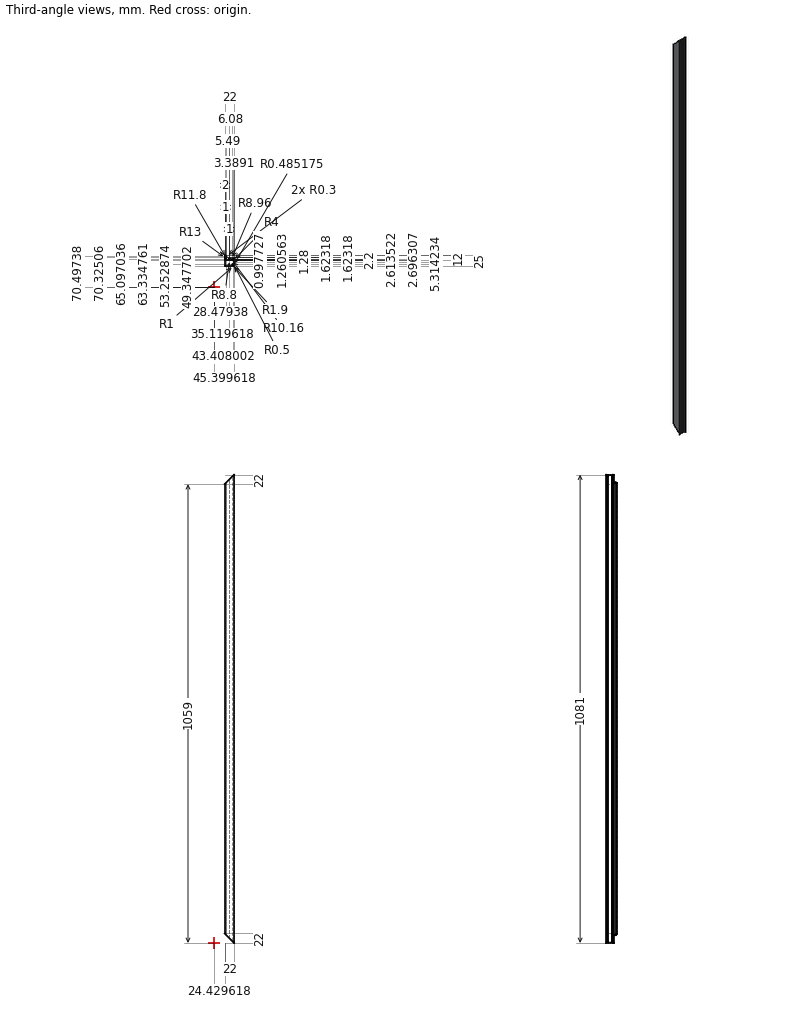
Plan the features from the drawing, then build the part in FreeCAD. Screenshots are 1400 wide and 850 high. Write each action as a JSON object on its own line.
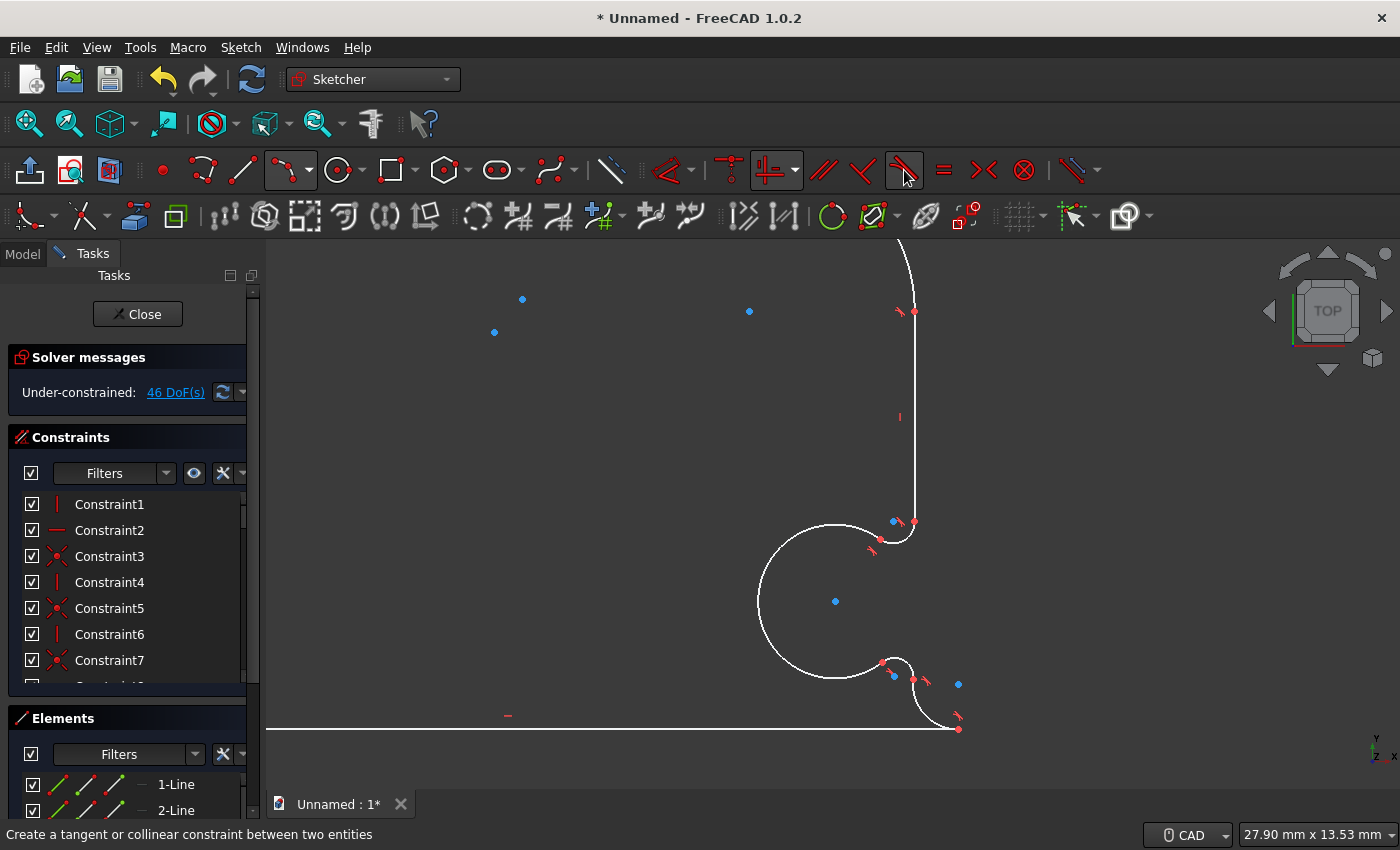
{"action": "scroll", "coordinate": [914, 686], "scroll_direction": "down", "scroll_amount": 5}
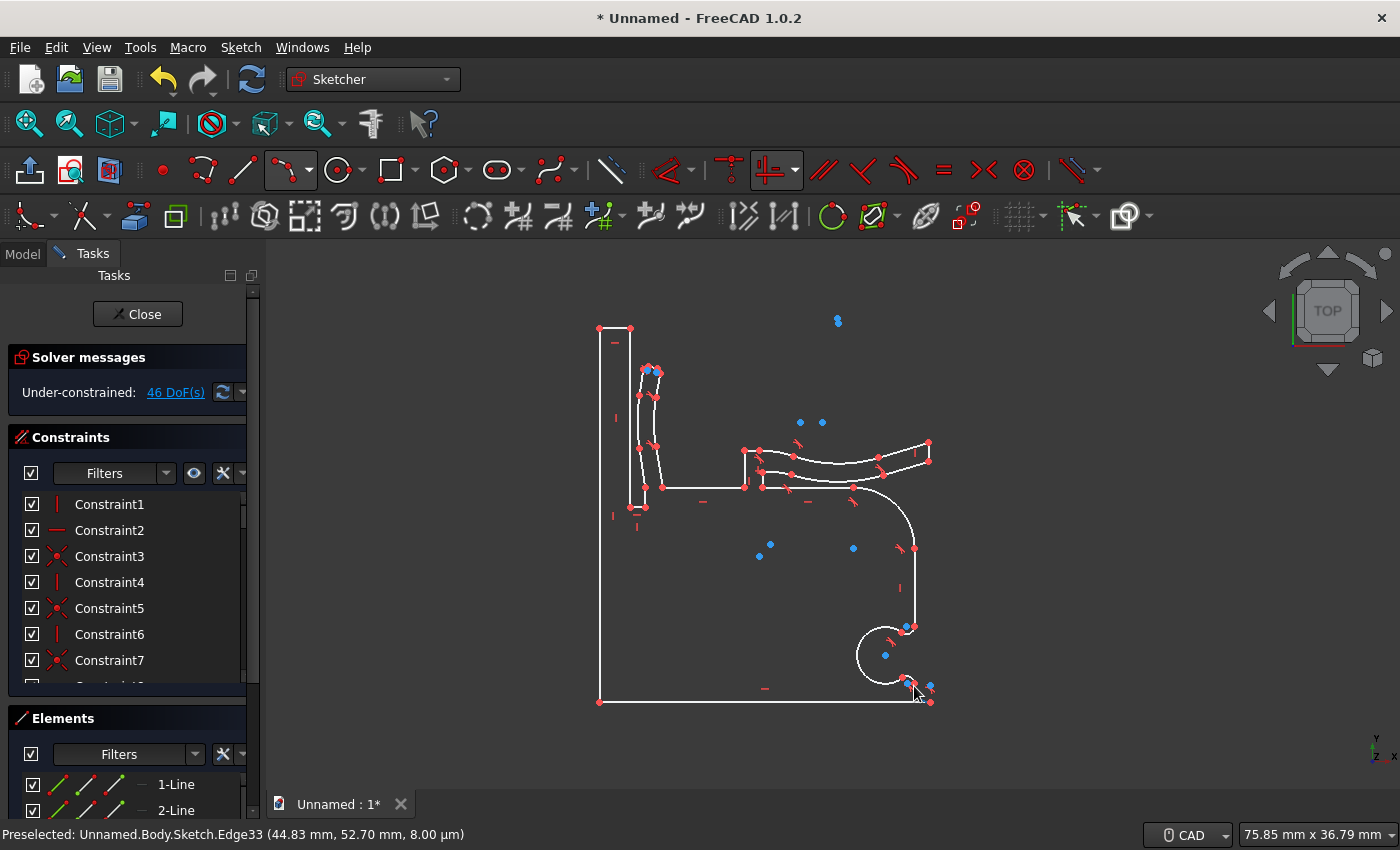
{"action": "scroll", "coordinate": [819, 481], "scroll_direction": "up", "scroll_amount": 4}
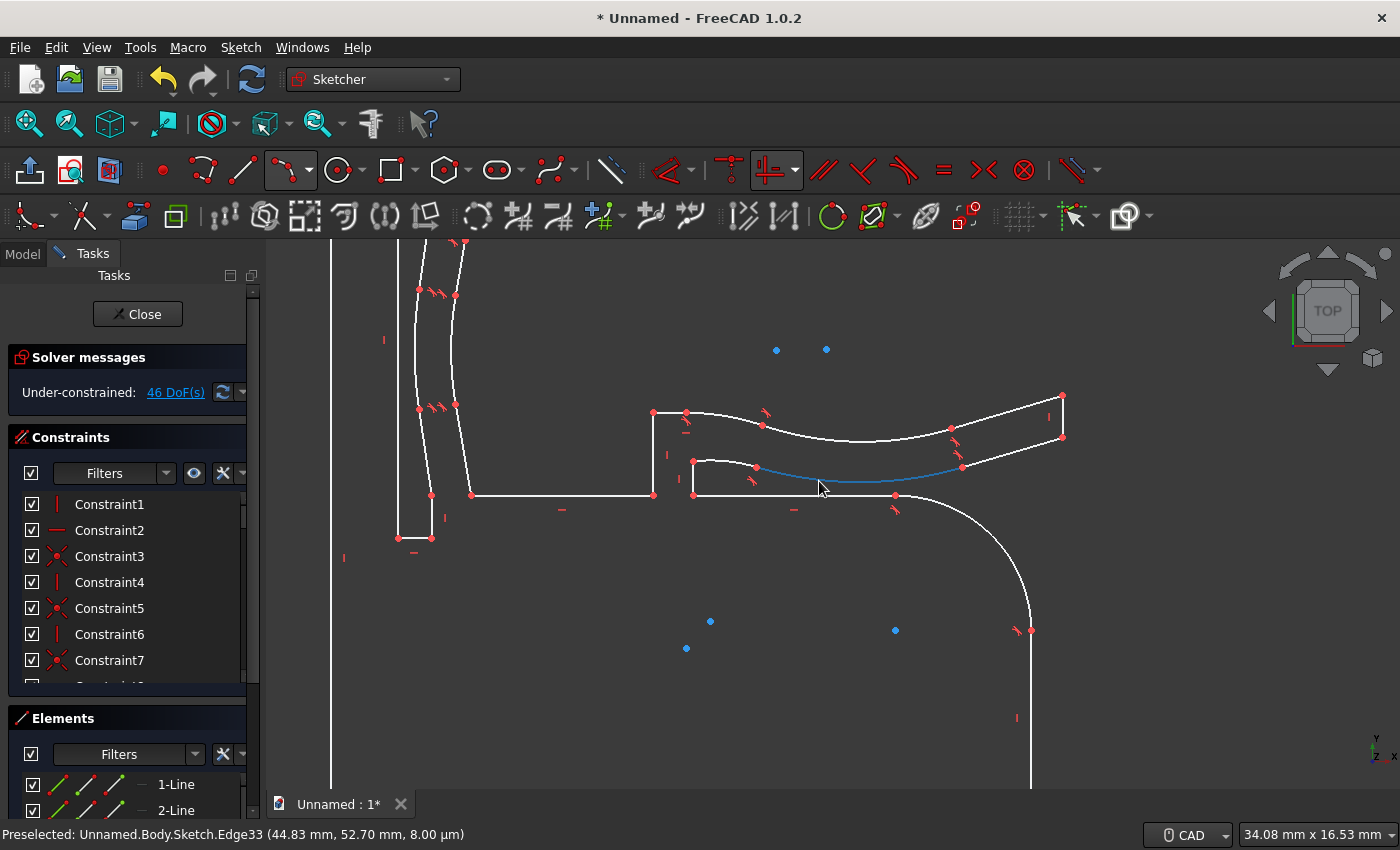
{"action": "left_click", "coordinate": [818, 480]}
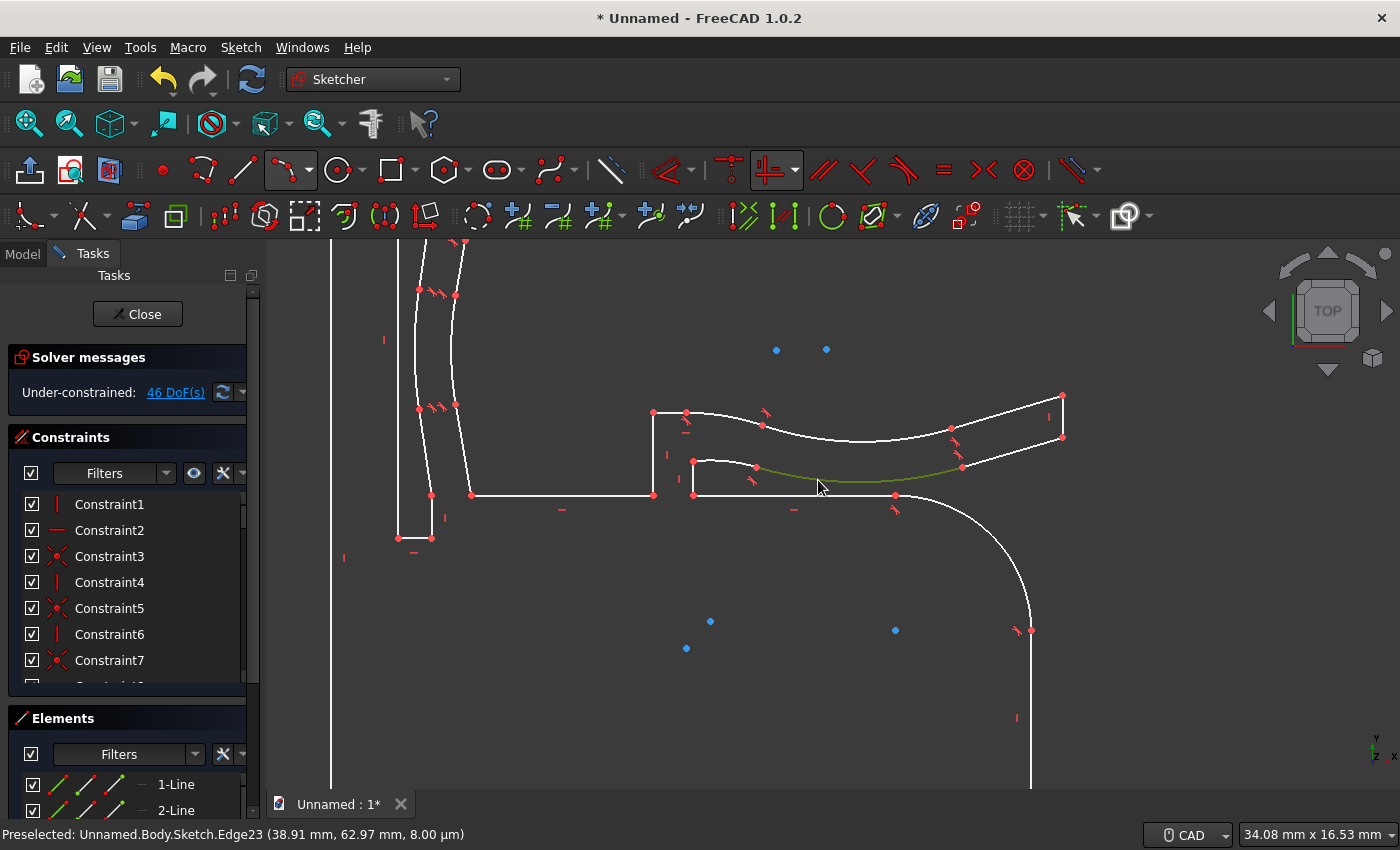
{"action": "left_click", "coordinate": [818, 439]}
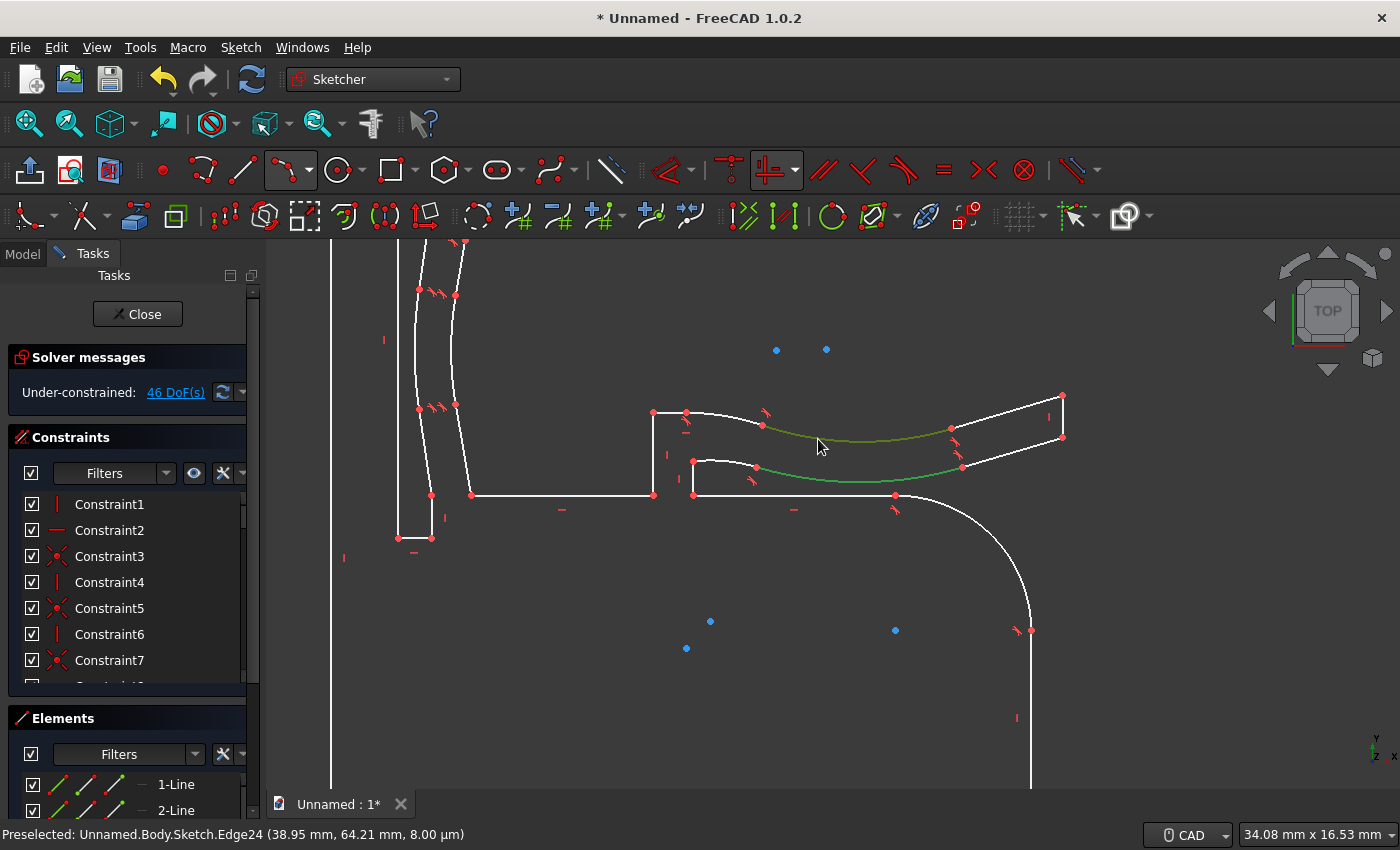
{"action": "left_click", "coordinate": [730, 170]}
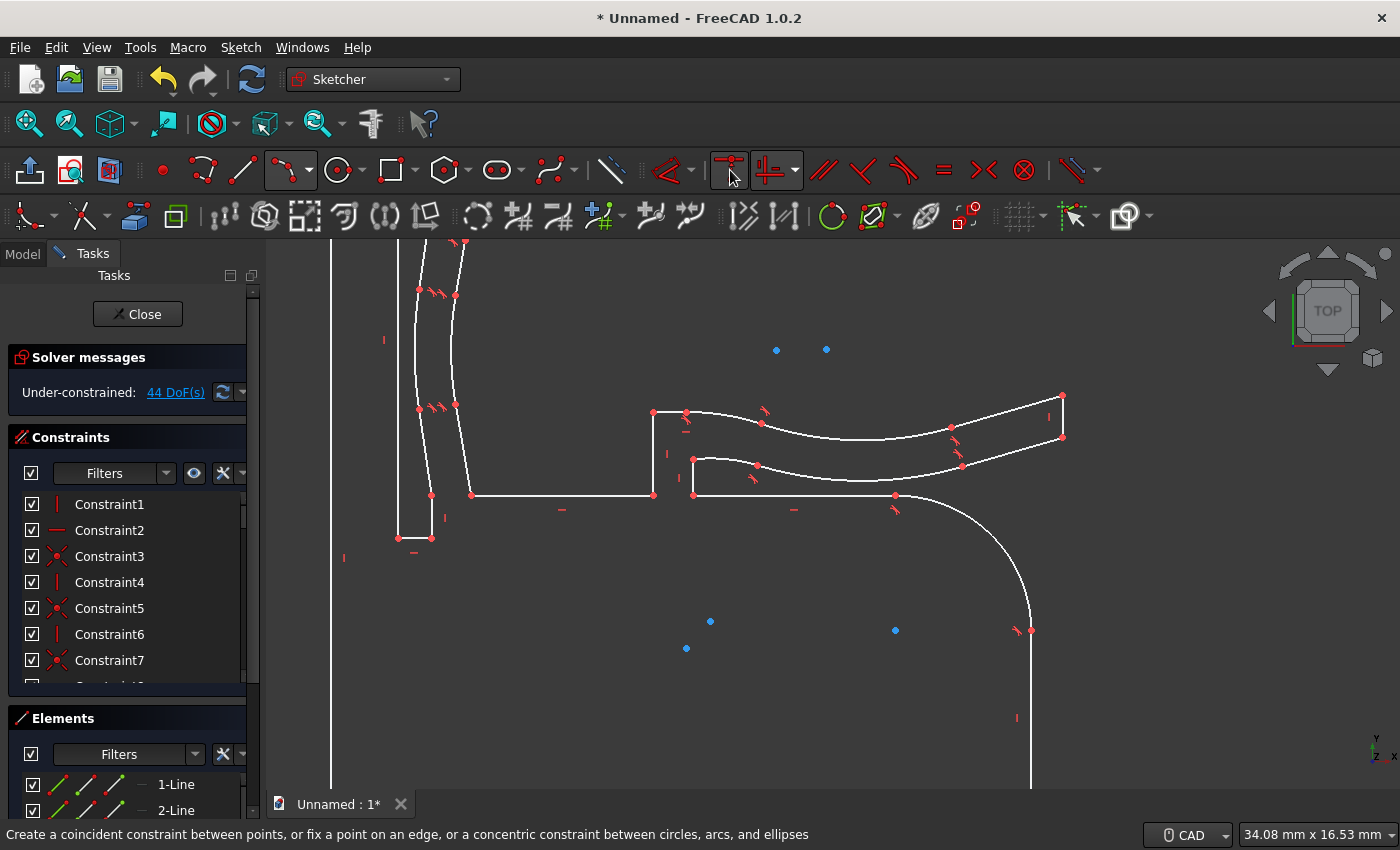
{"action": "left_click", "coordinate": [739, 461]}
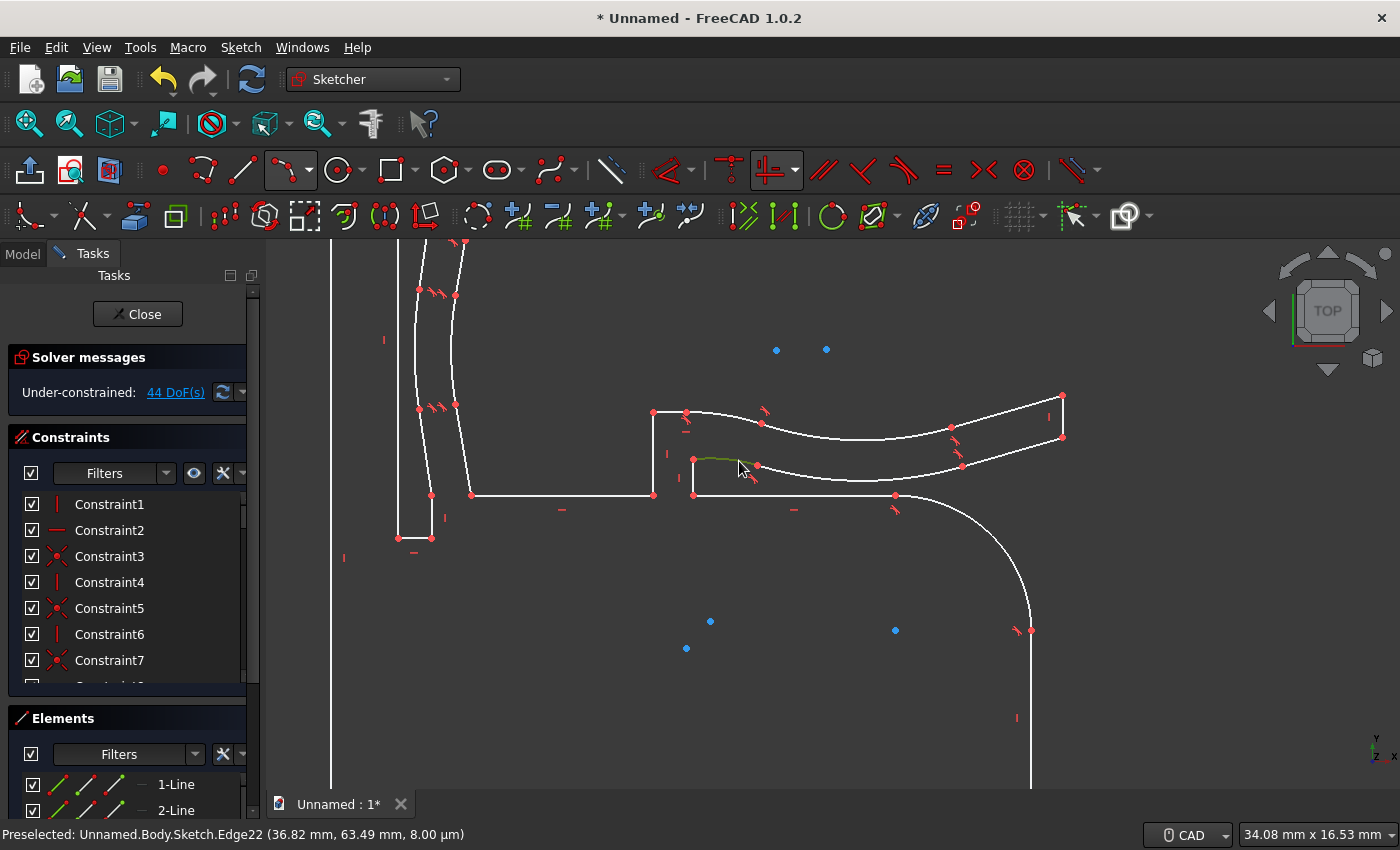
{"action": "left_click", "coordinate": [739, 418]}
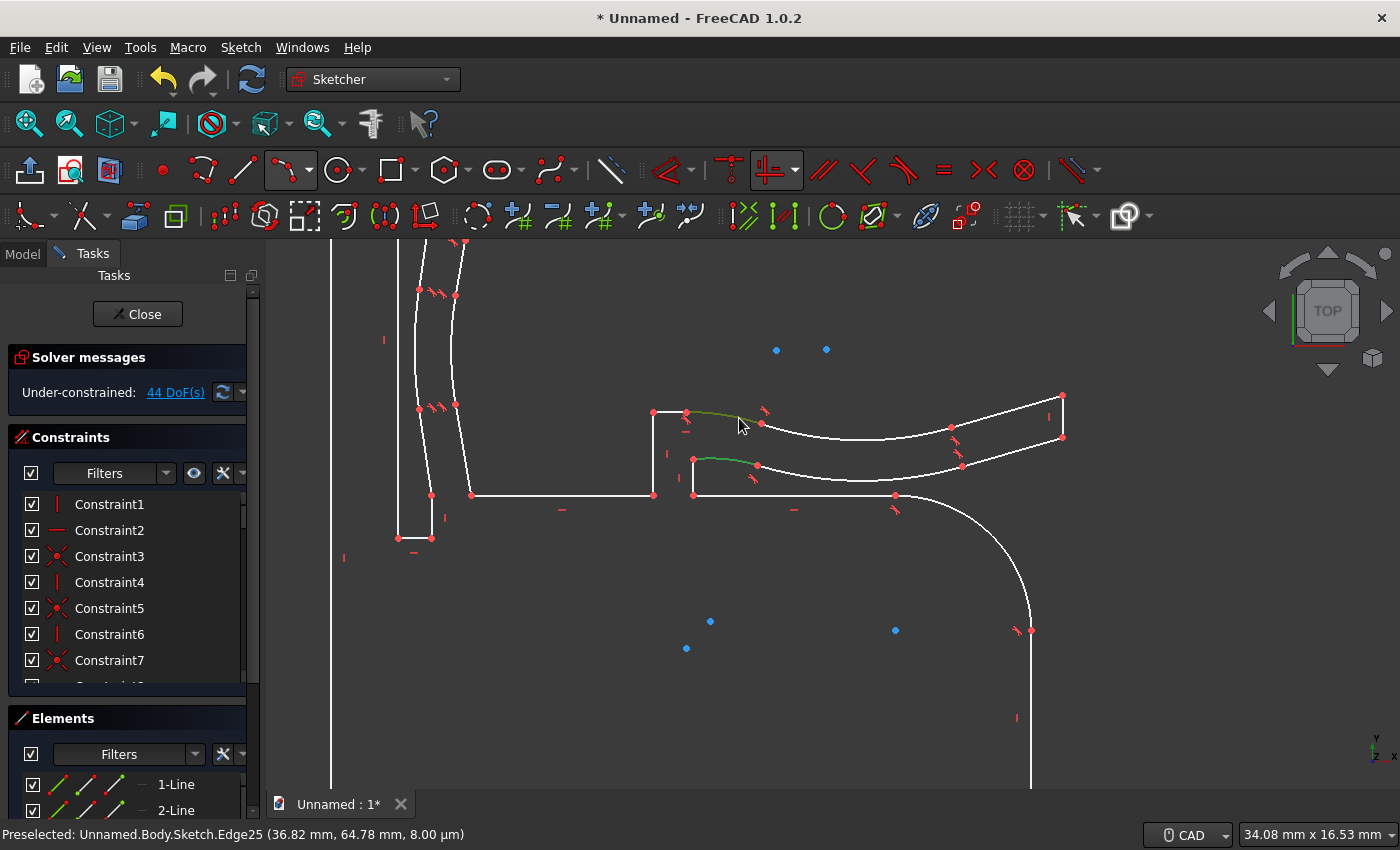
{"action": "left_click", "coordinate": [730, 170]}